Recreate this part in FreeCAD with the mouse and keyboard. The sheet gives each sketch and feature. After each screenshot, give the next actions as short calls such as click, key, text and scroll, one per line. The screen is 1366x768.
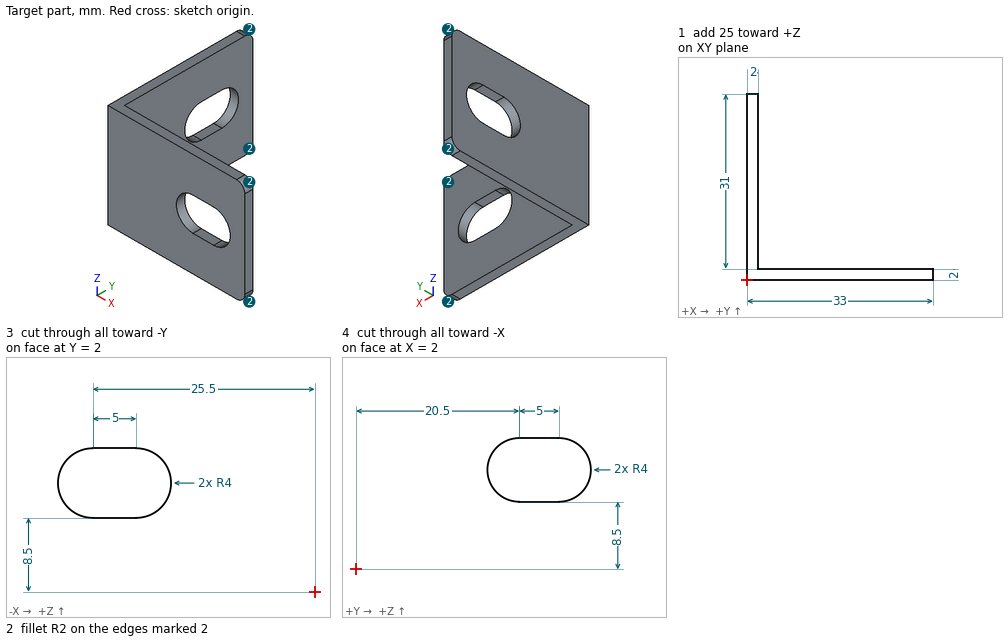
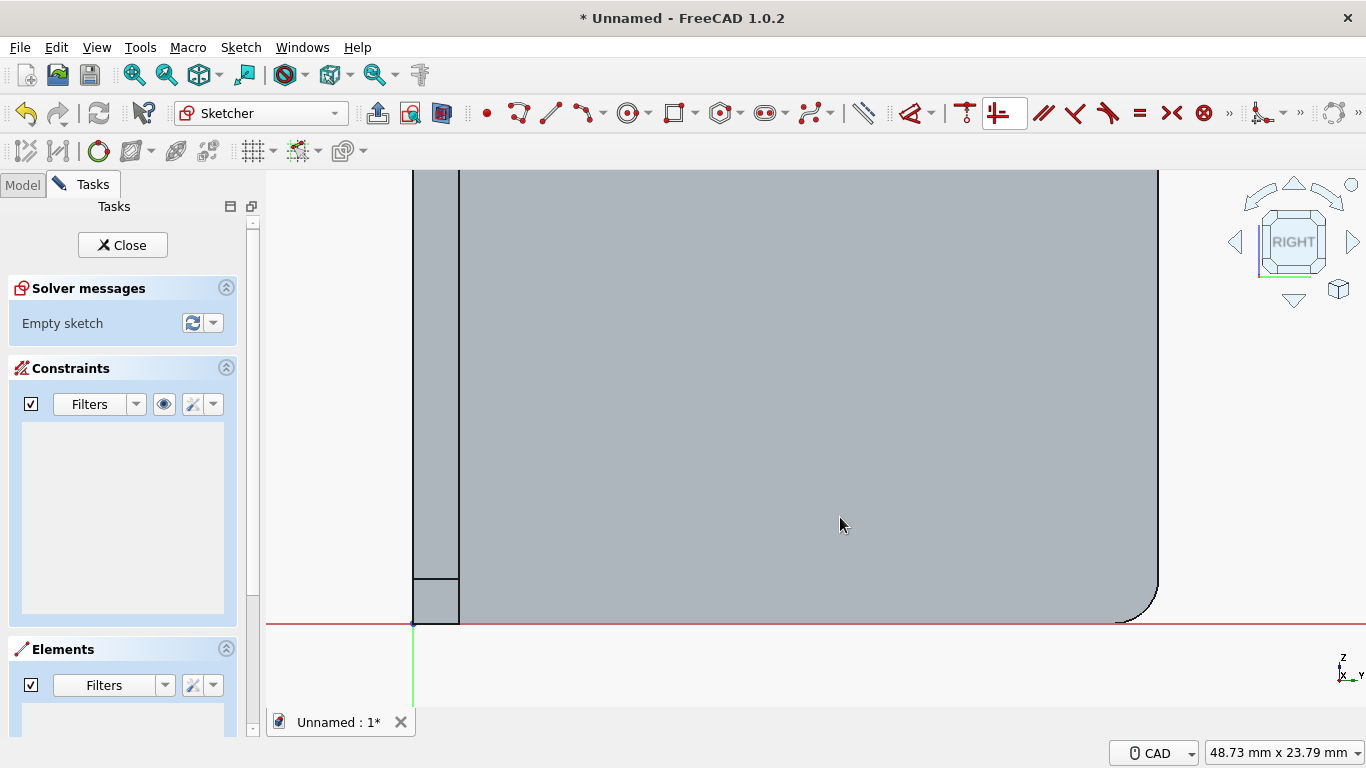
click(876, 342)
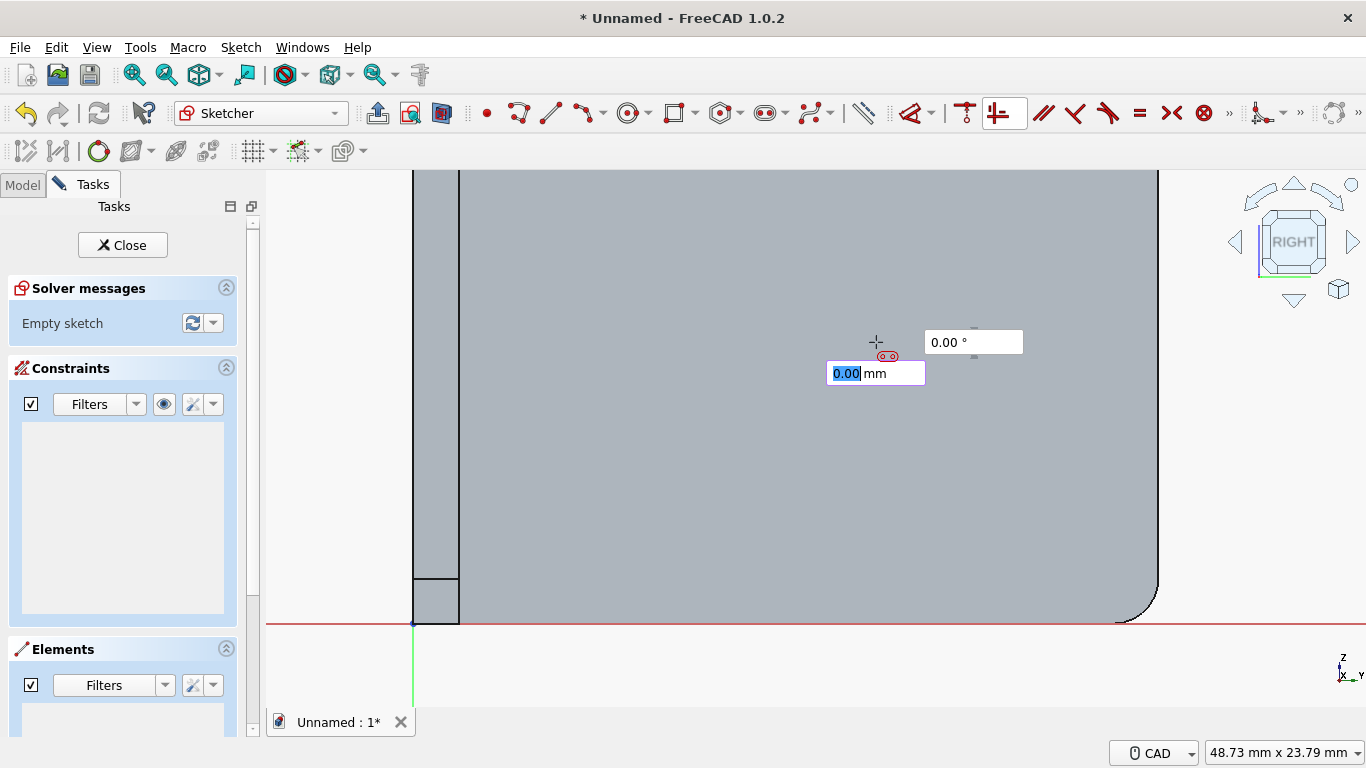
click(989, 342)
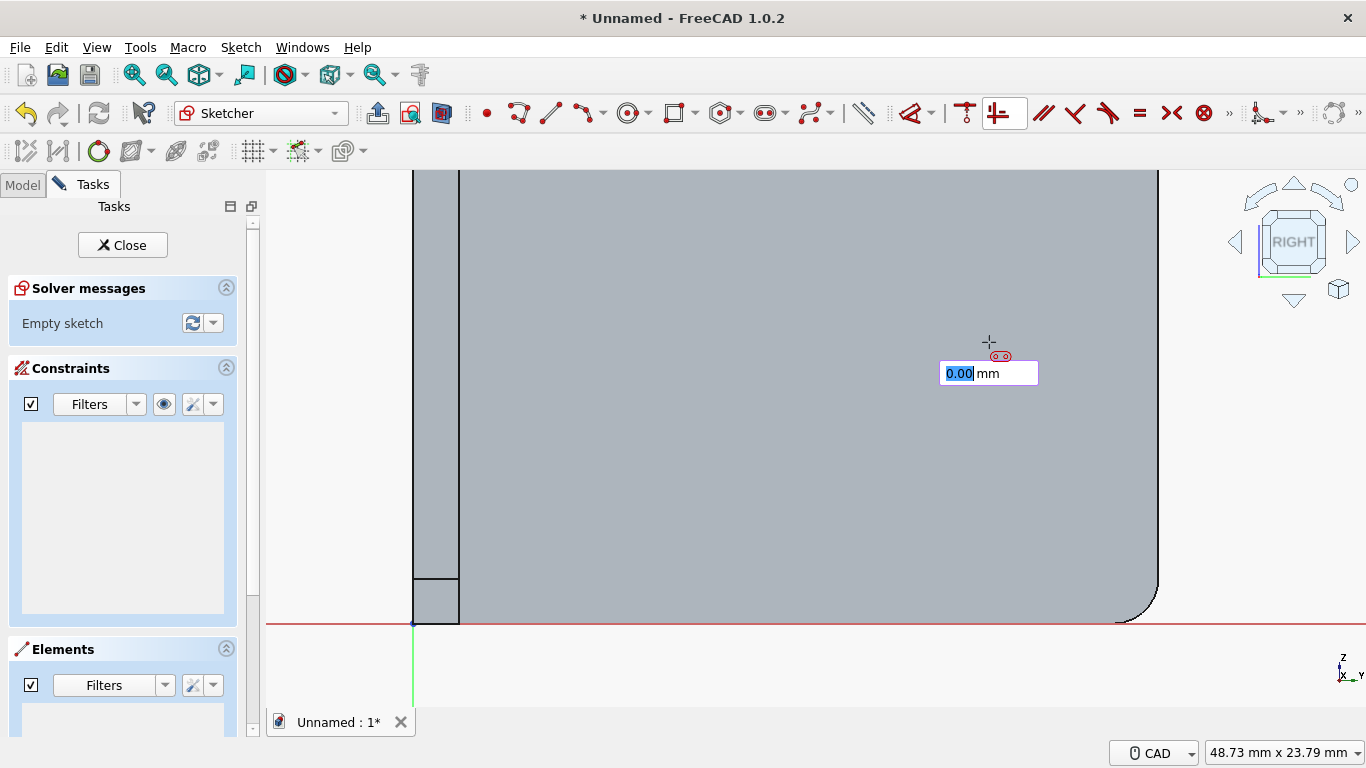
click(933, 432)
key(Escape)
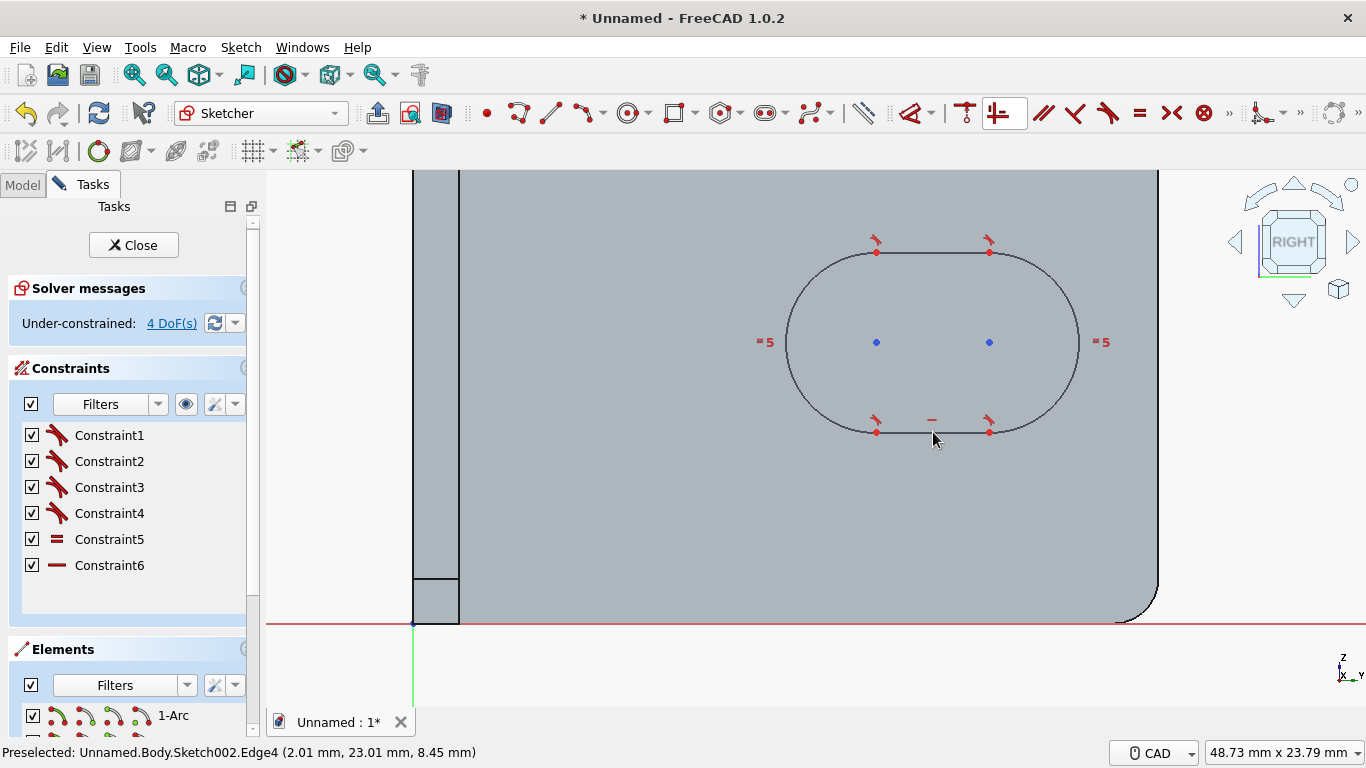
click(803, 290)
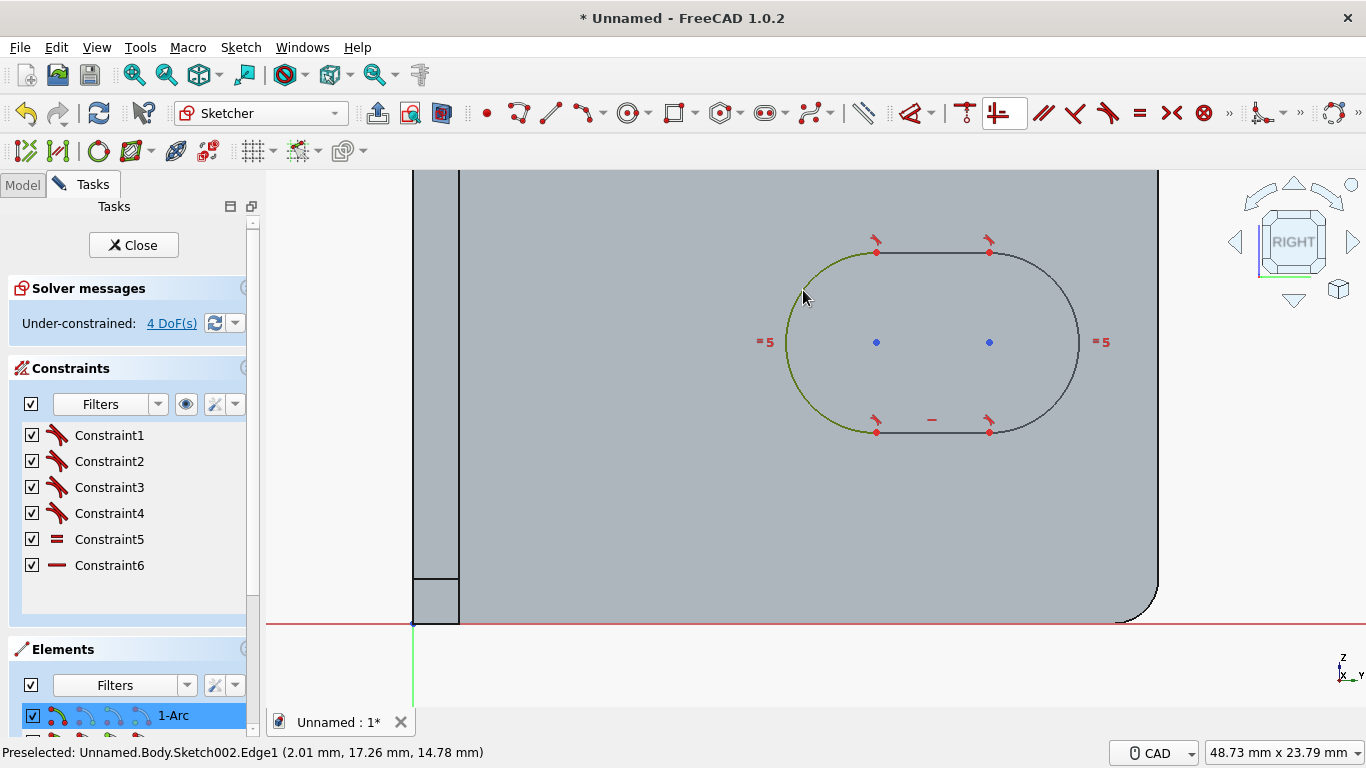
key(k)
key(r)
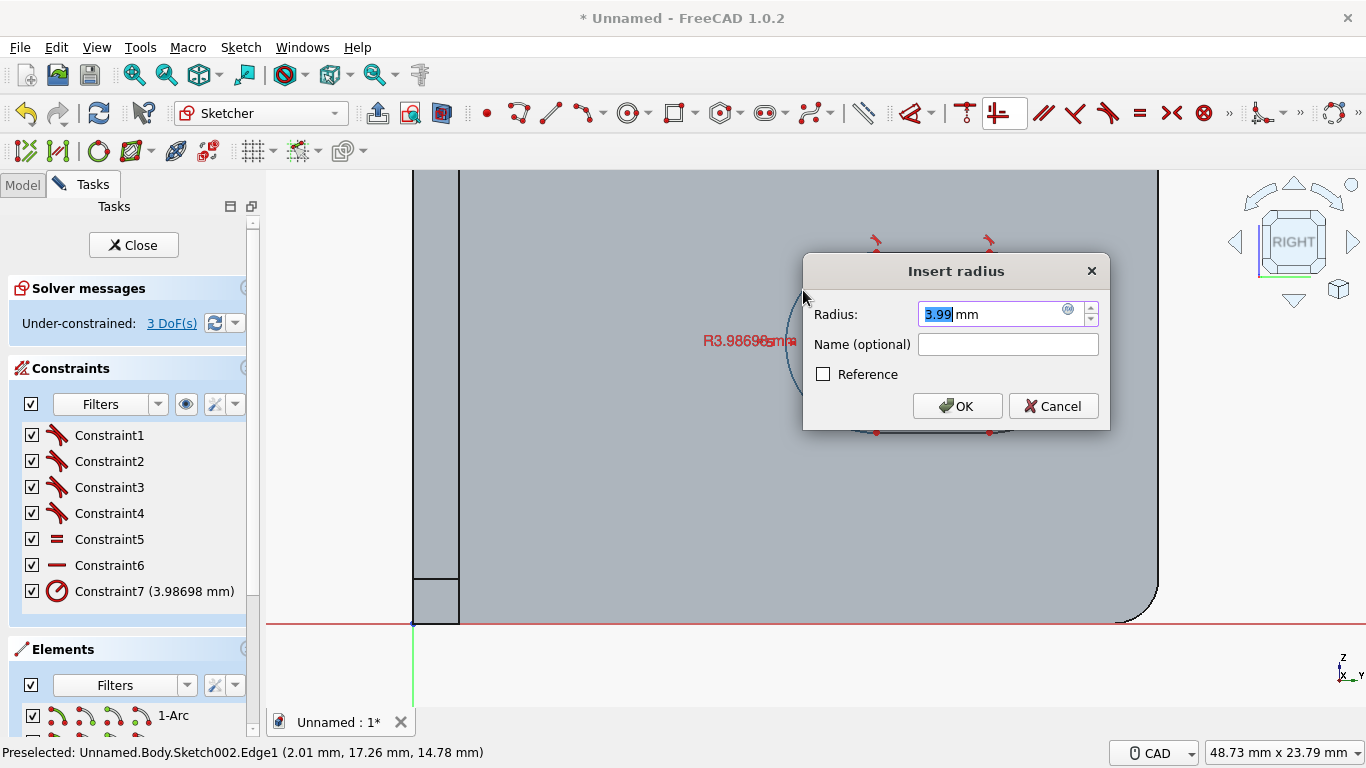
text(4)
key(Return)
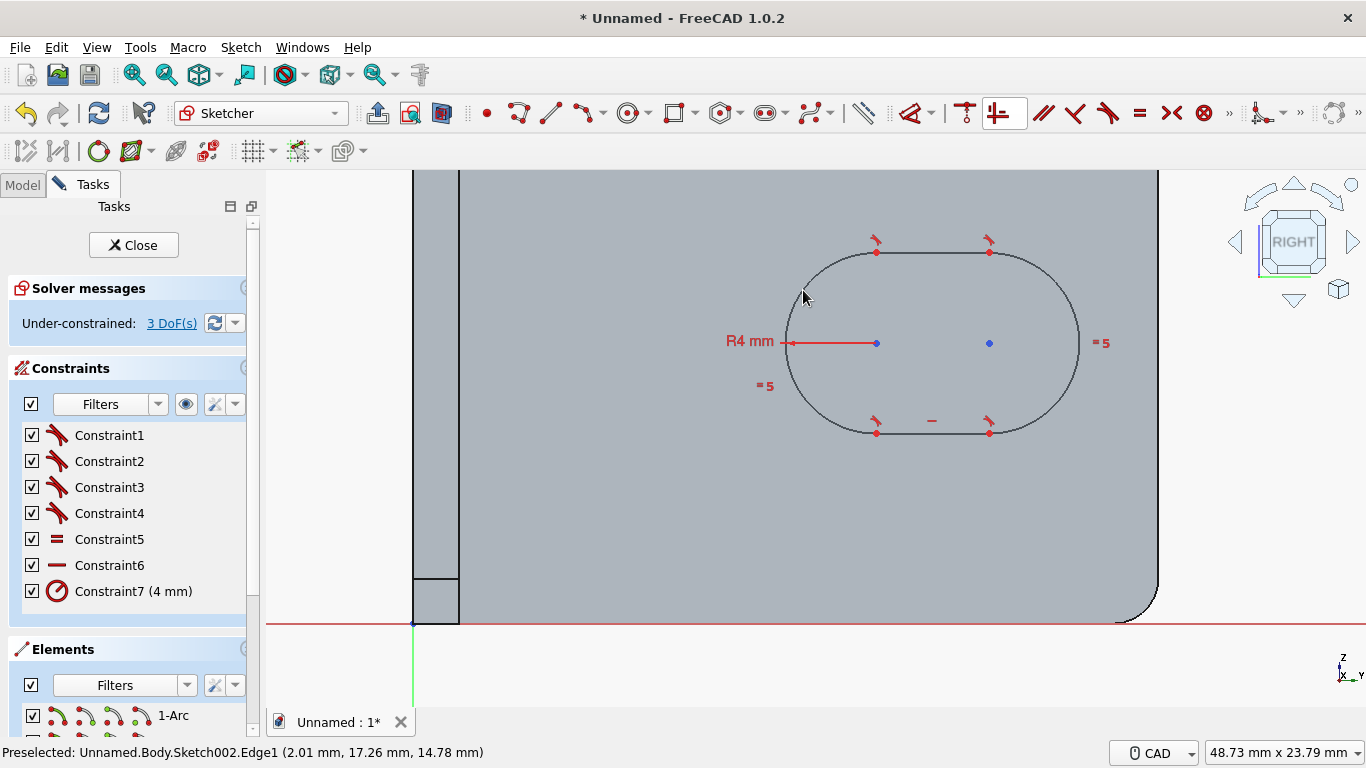
click(910, 253)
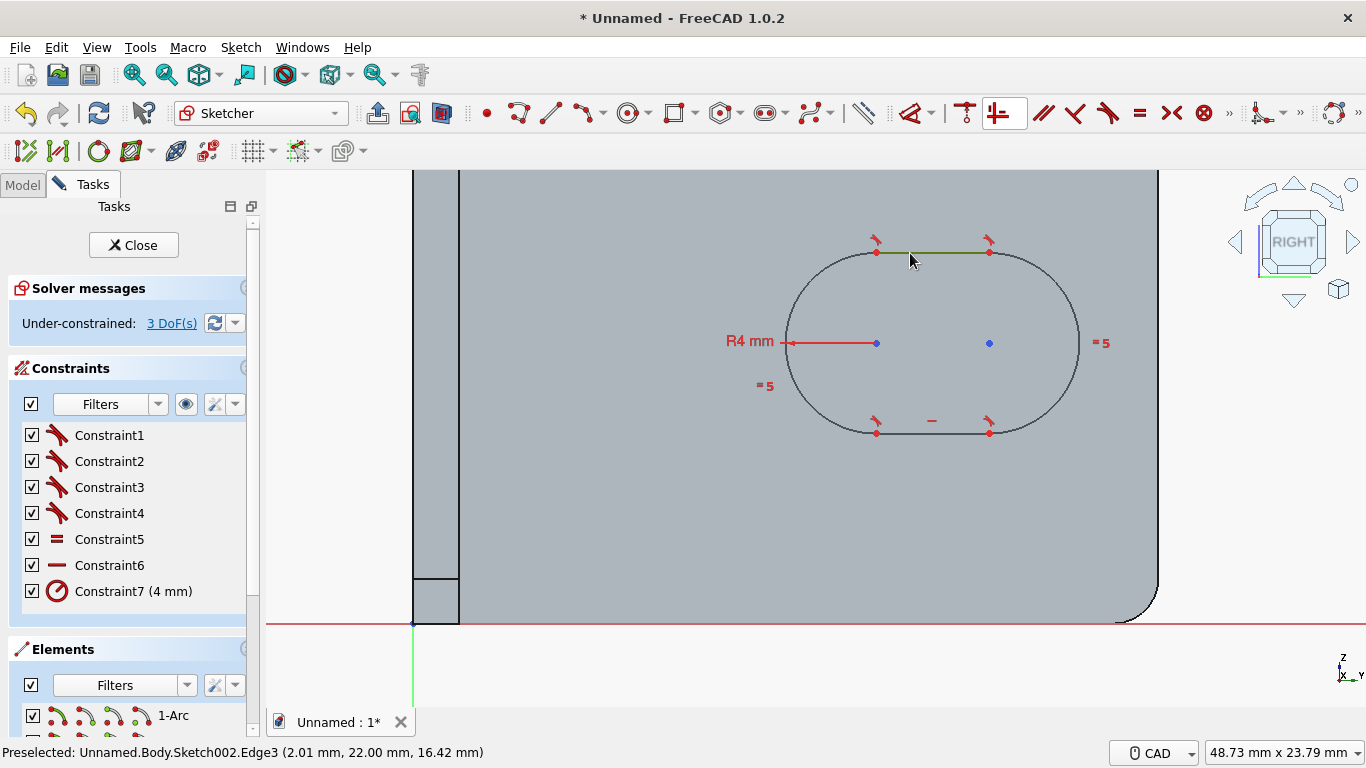
key(l)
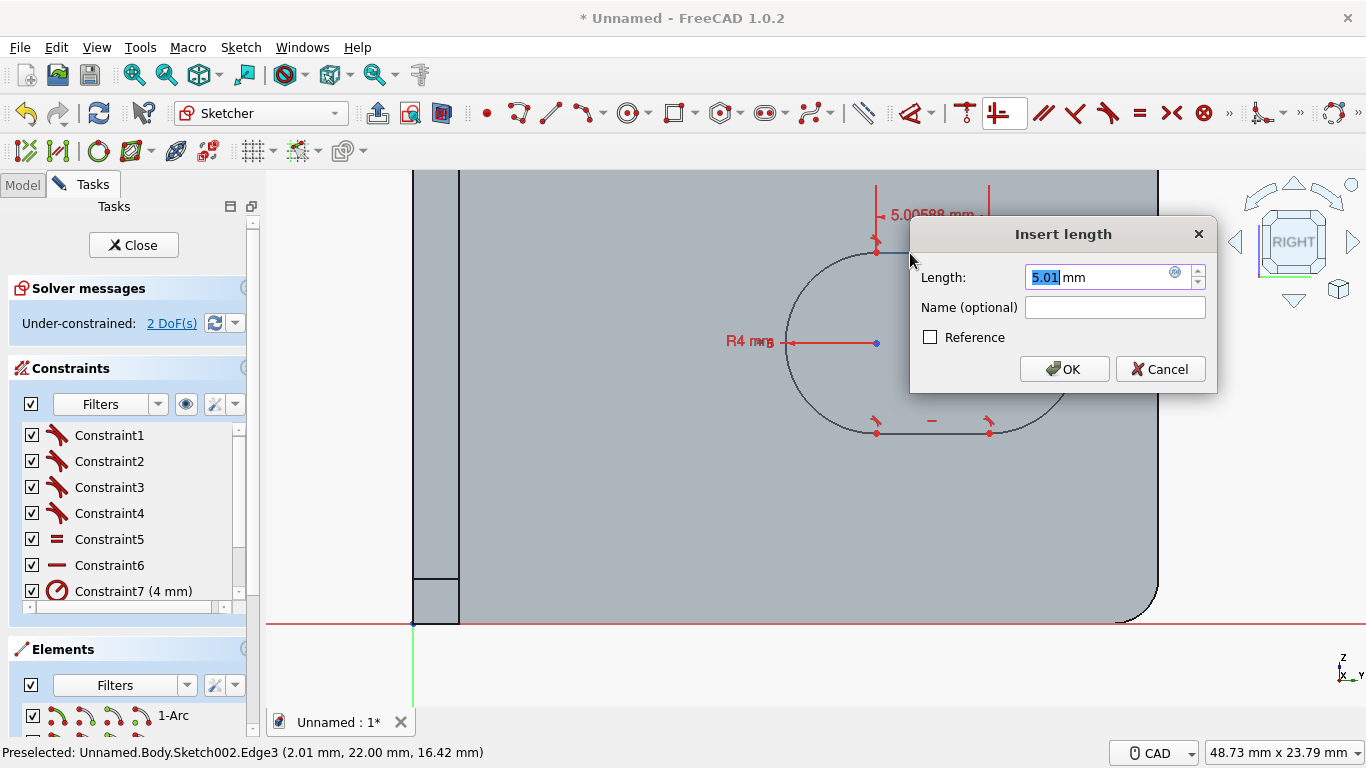
text(5)
key(Return)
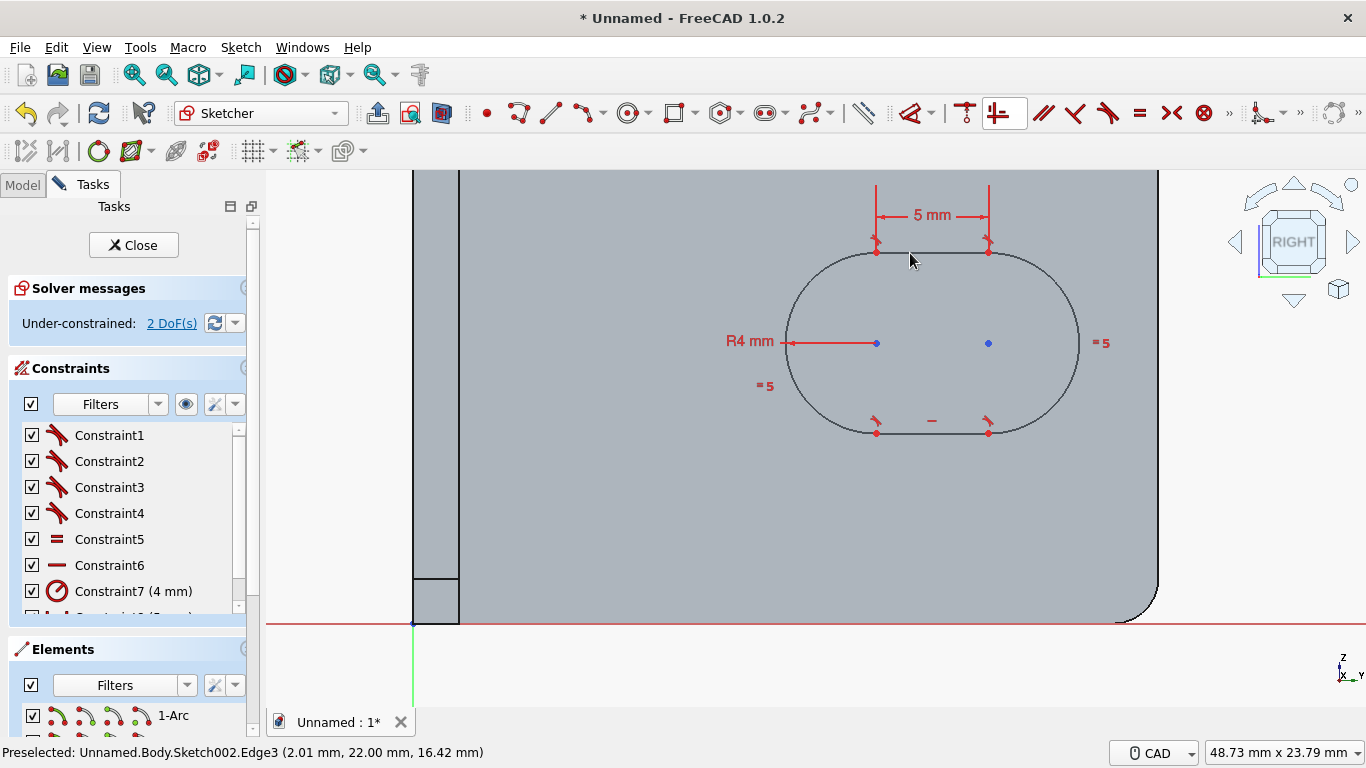
click(876, 434)